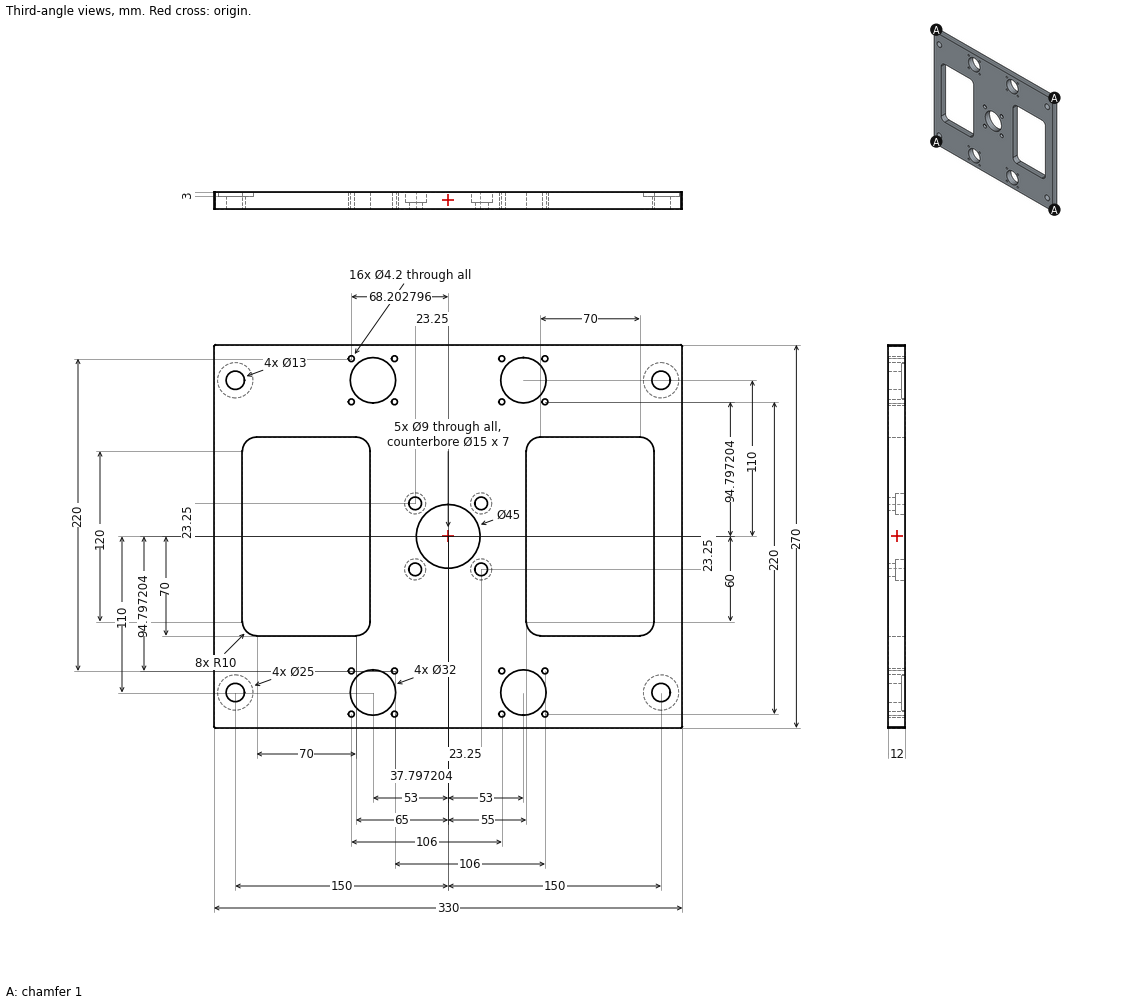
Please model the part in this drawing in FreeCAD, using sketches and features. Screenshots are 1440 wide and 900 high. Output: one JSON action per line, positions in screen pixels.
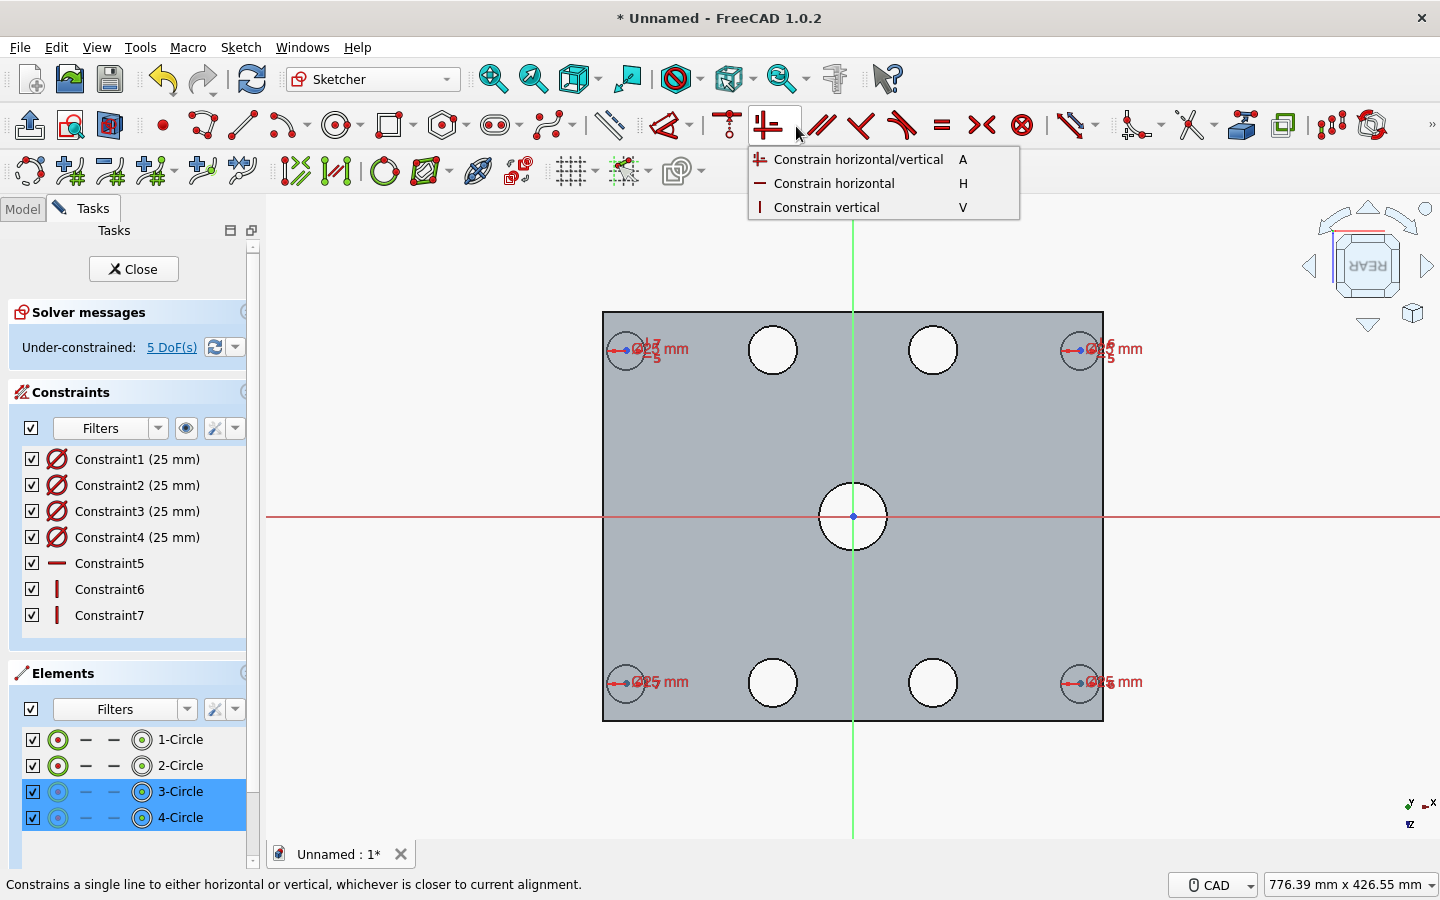
{"action": "left_click", "coordinate": [884, 183]}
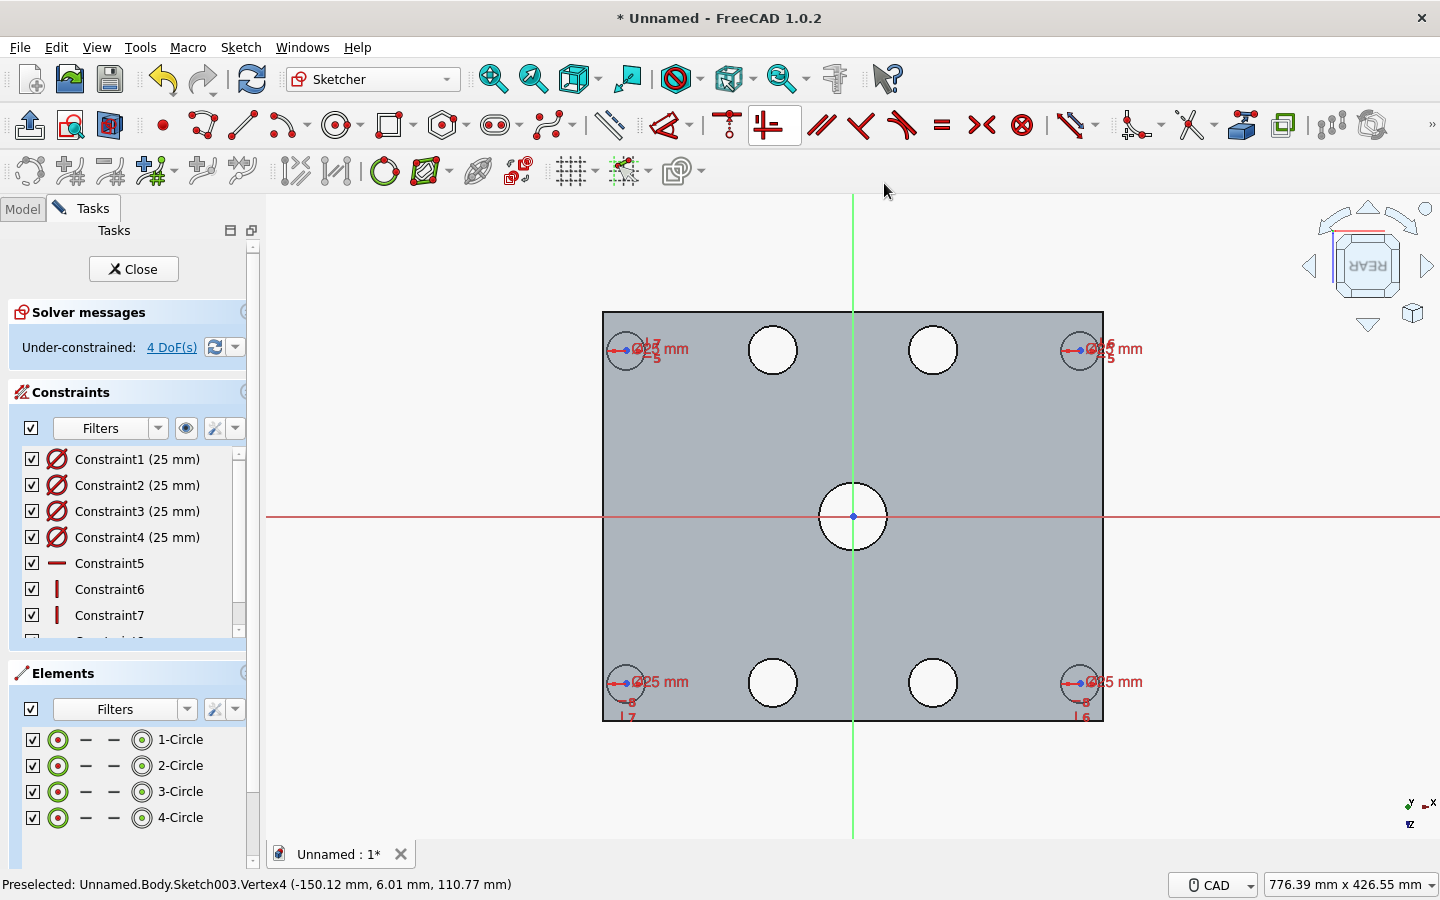
{"action": "left_click", "coordinate": [664, 126]}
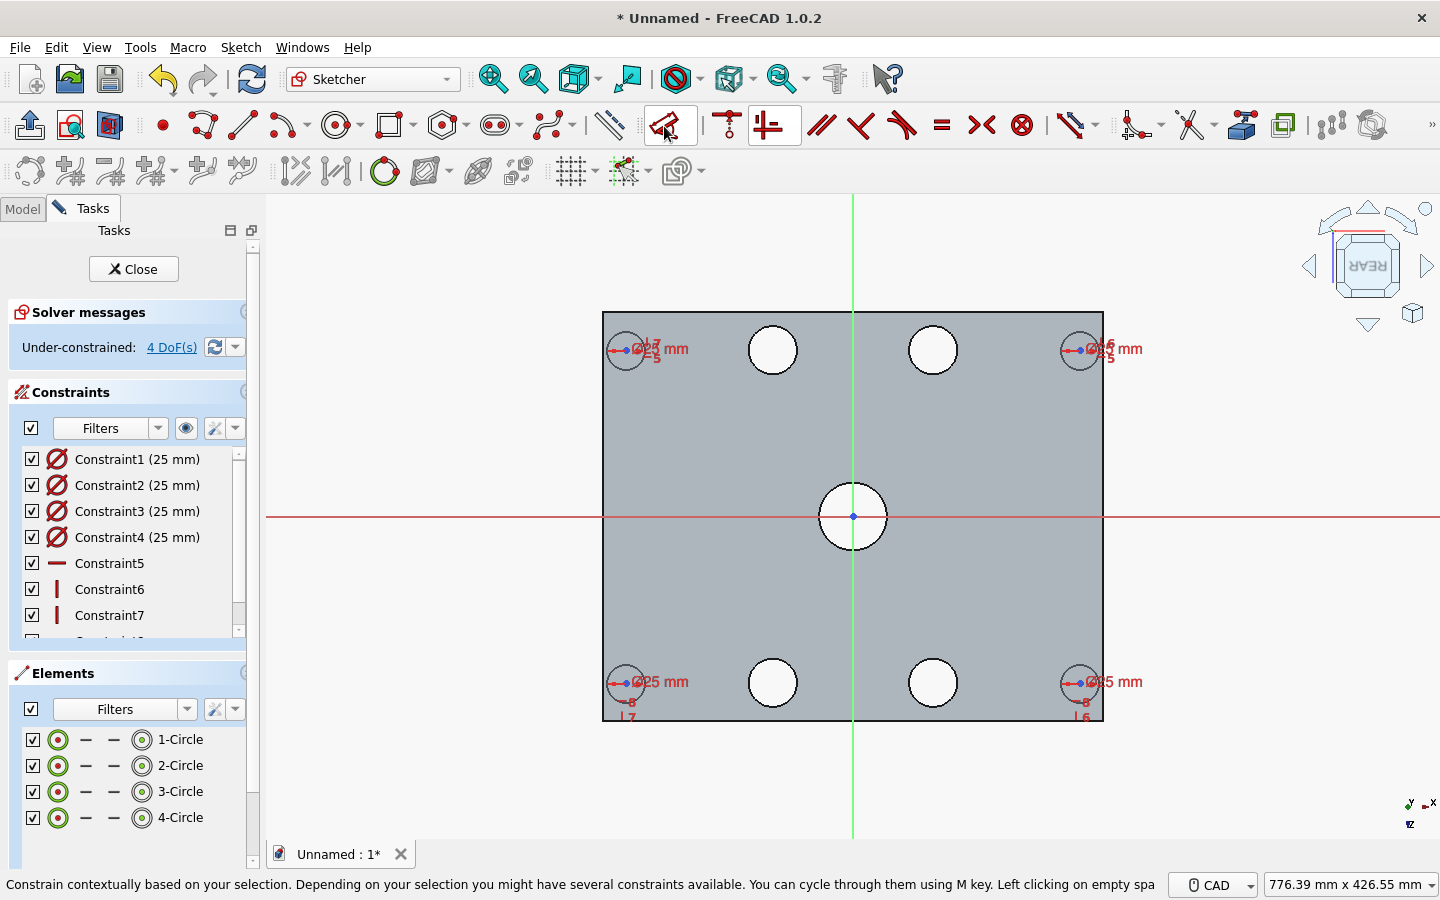
{"action": "left_click", "coordinate": [626, 351]}
{"action": "left_click", "coordinate": [740, 317]}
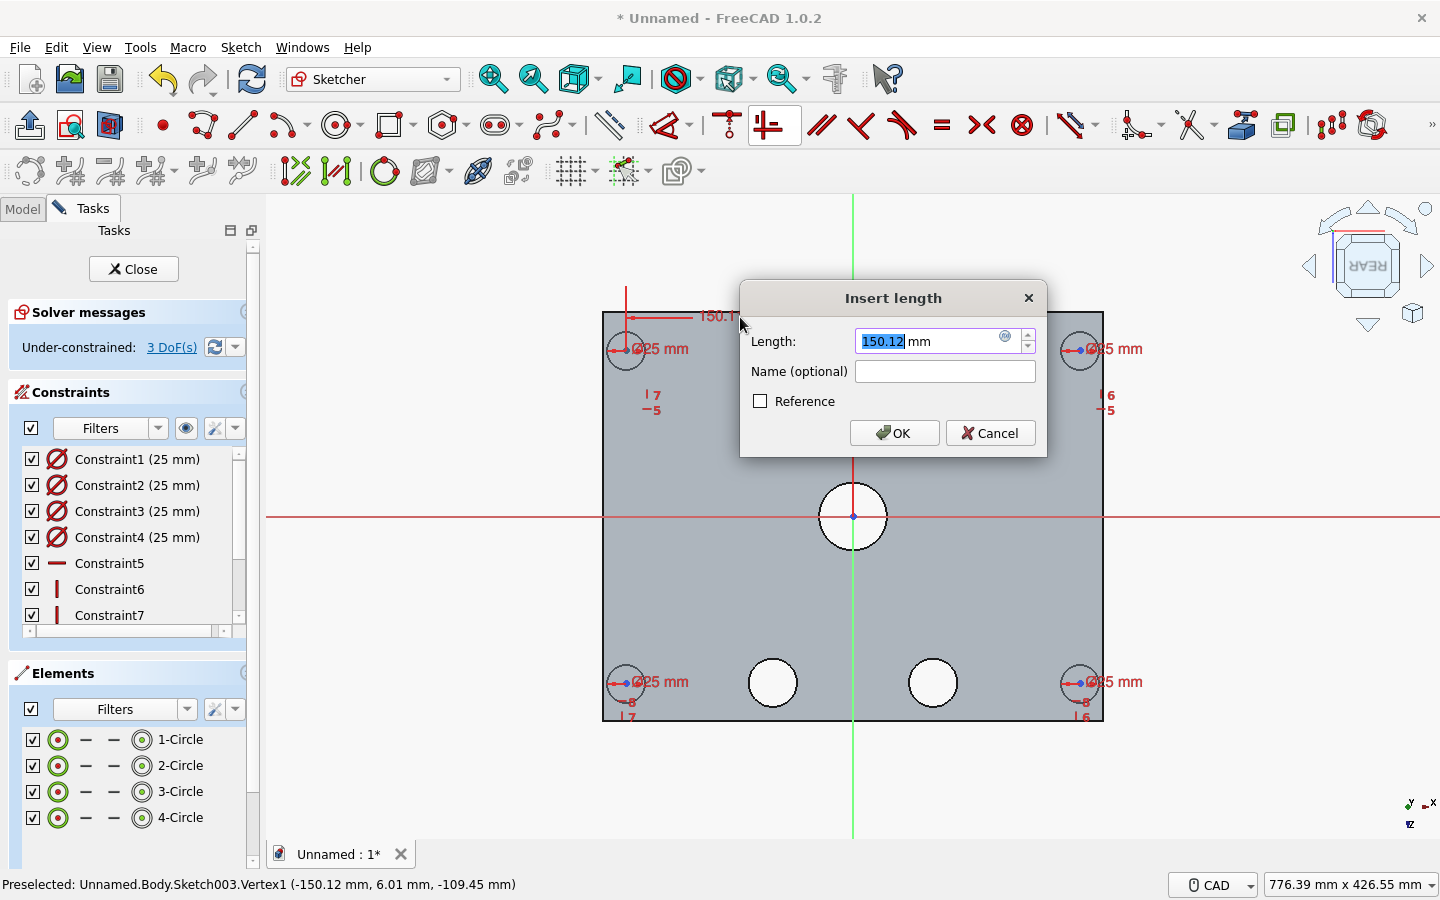
{"action": "type", "text": "150"}
{"action": "key", "text": "Return"}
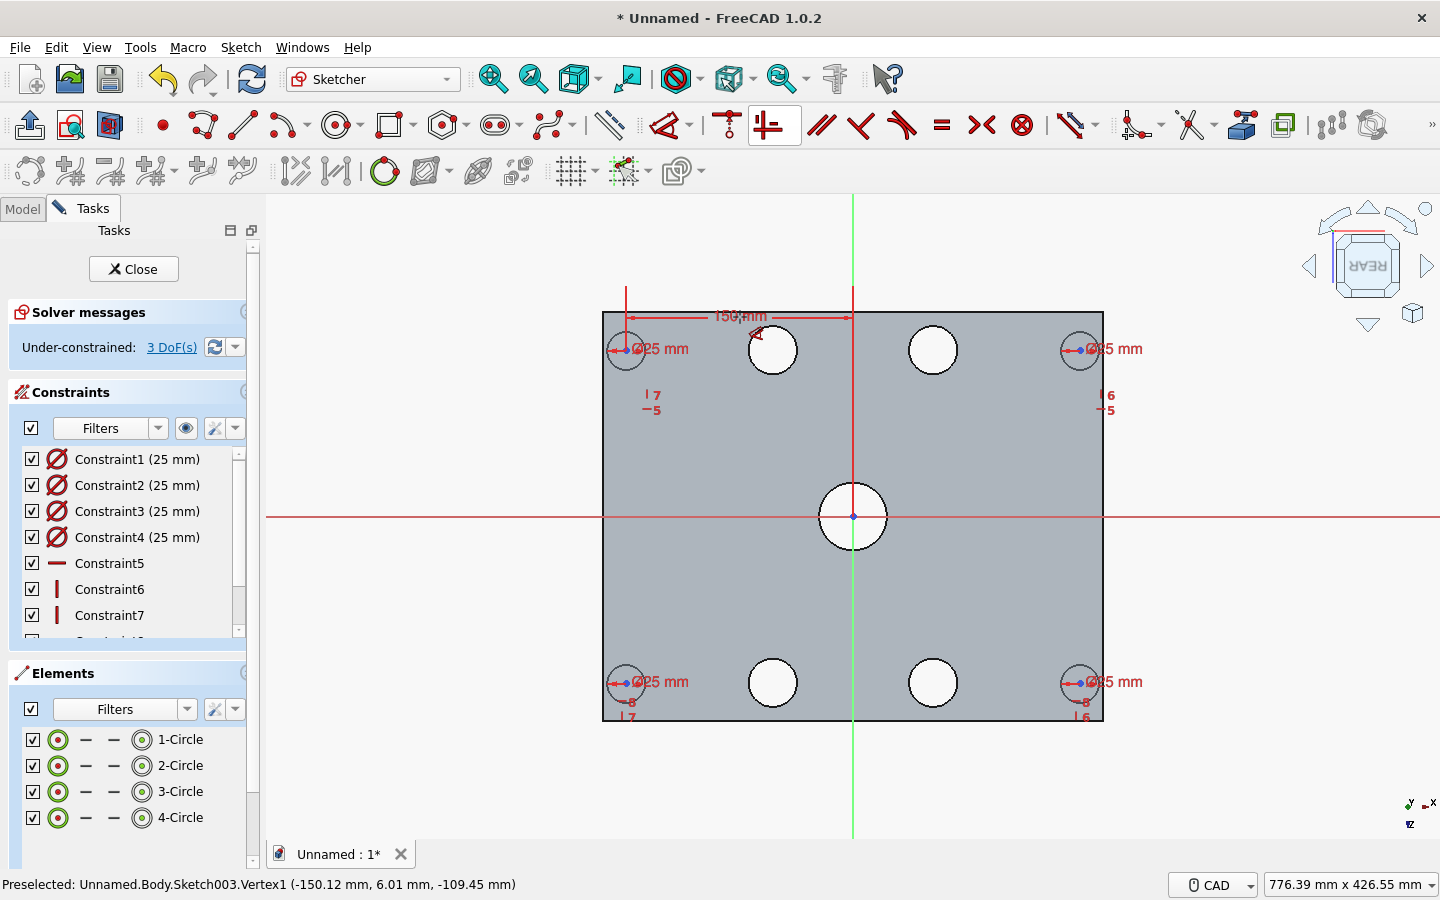
{"action": "left_click", "coordinate": [626, 351]}
{"action": "left_click", "coordinate": [592, 434]}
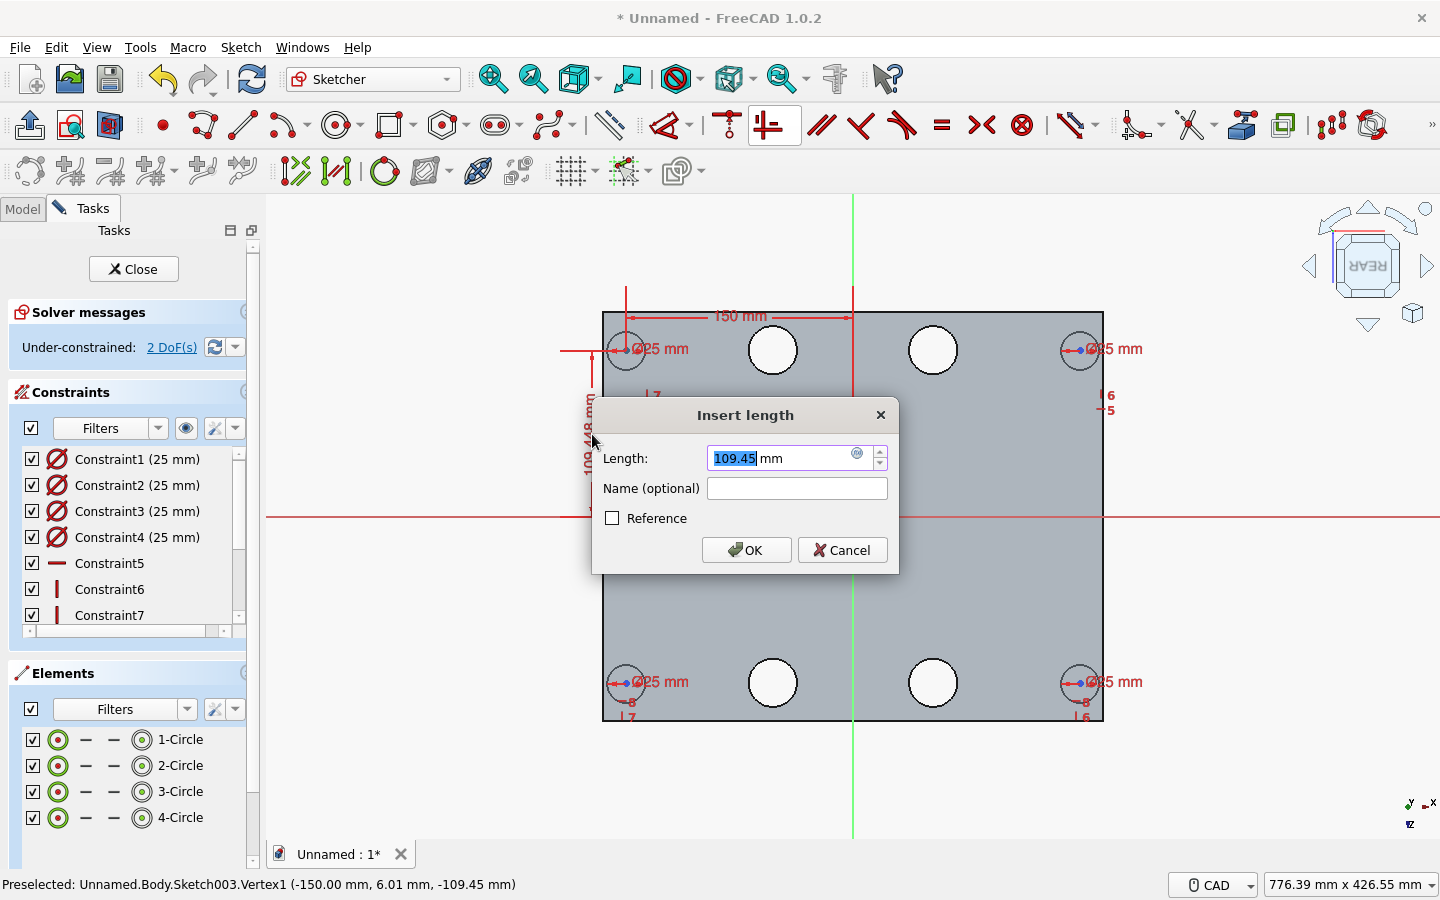
{"action": "type", "text": "110"}
{"action": "key", "text": "Return"}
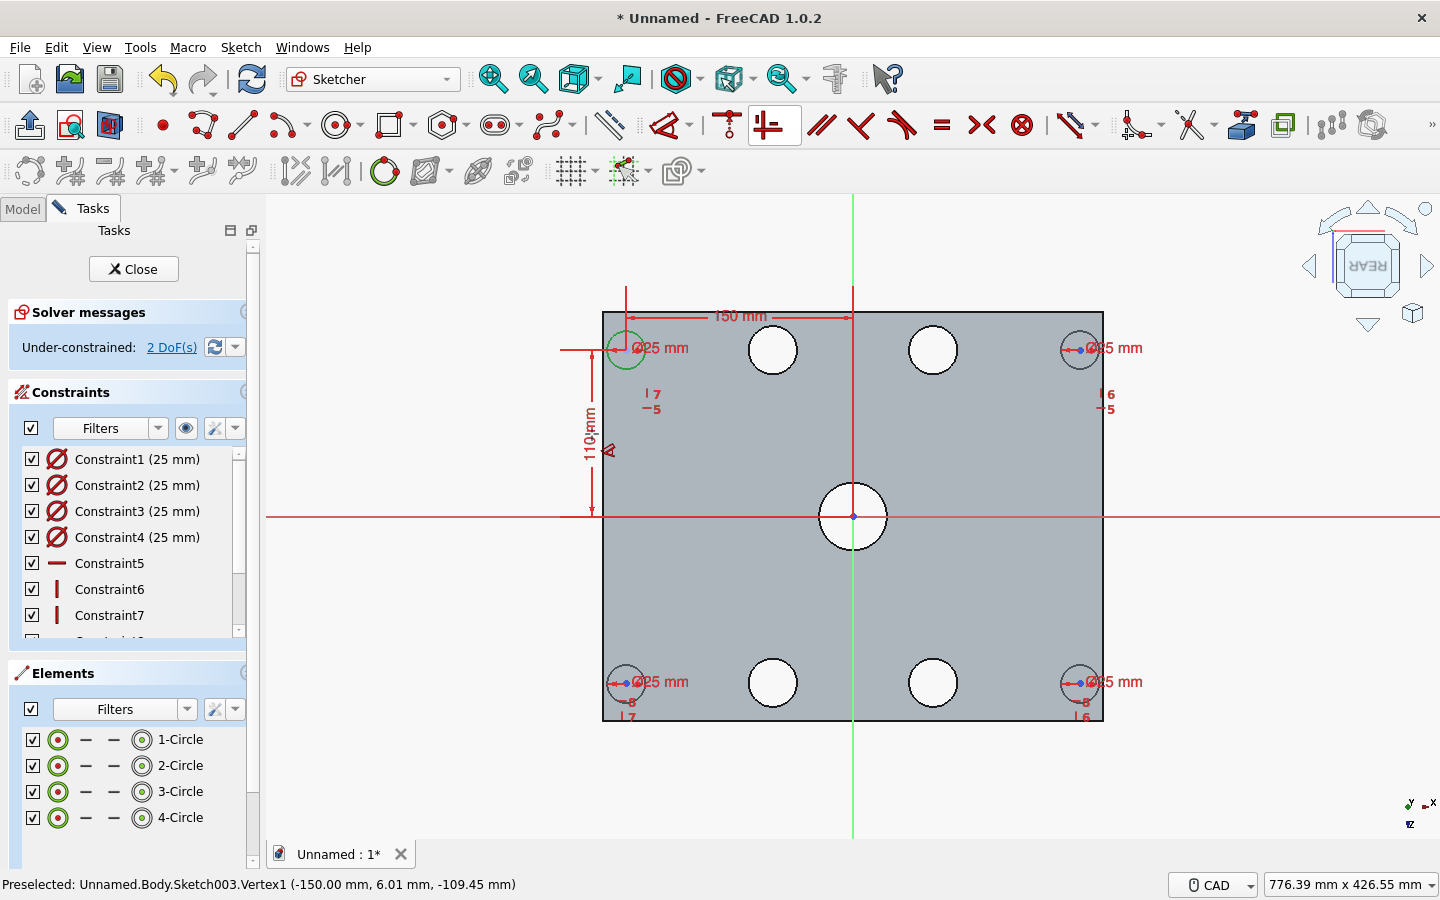
{"action": "left_click", "coordinate": [1080, 350]}
{"action": "left_click", "coordinate": [966, 316]}